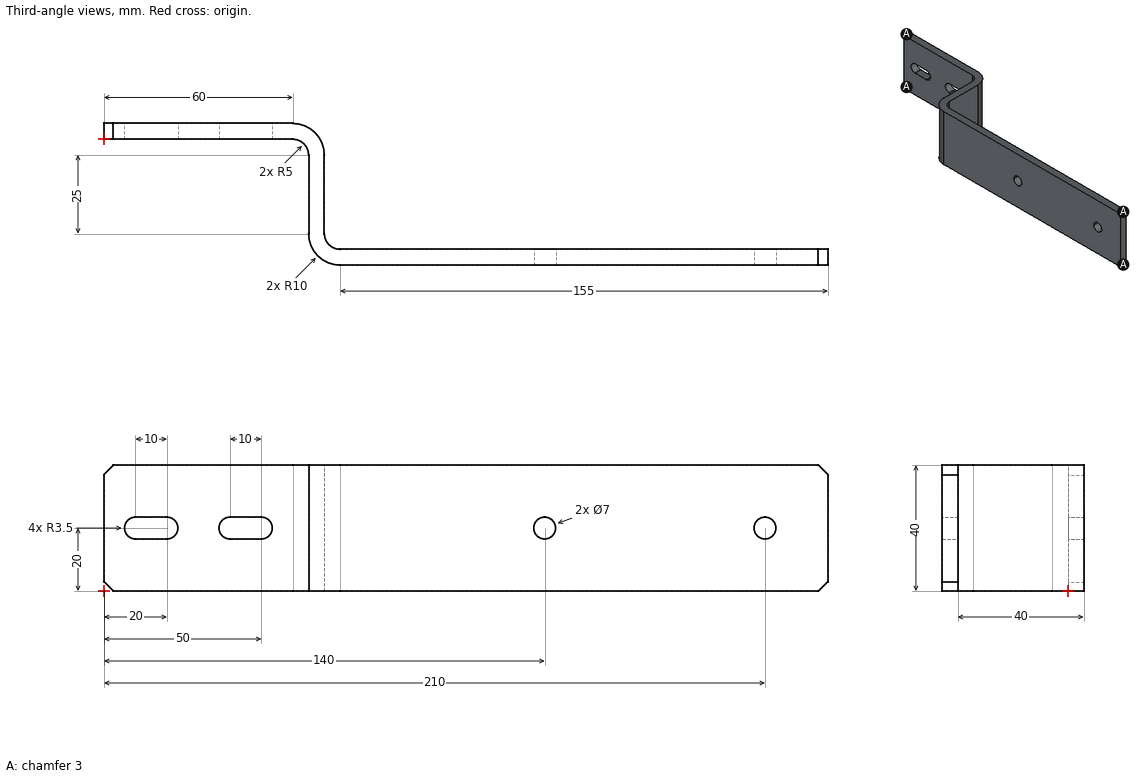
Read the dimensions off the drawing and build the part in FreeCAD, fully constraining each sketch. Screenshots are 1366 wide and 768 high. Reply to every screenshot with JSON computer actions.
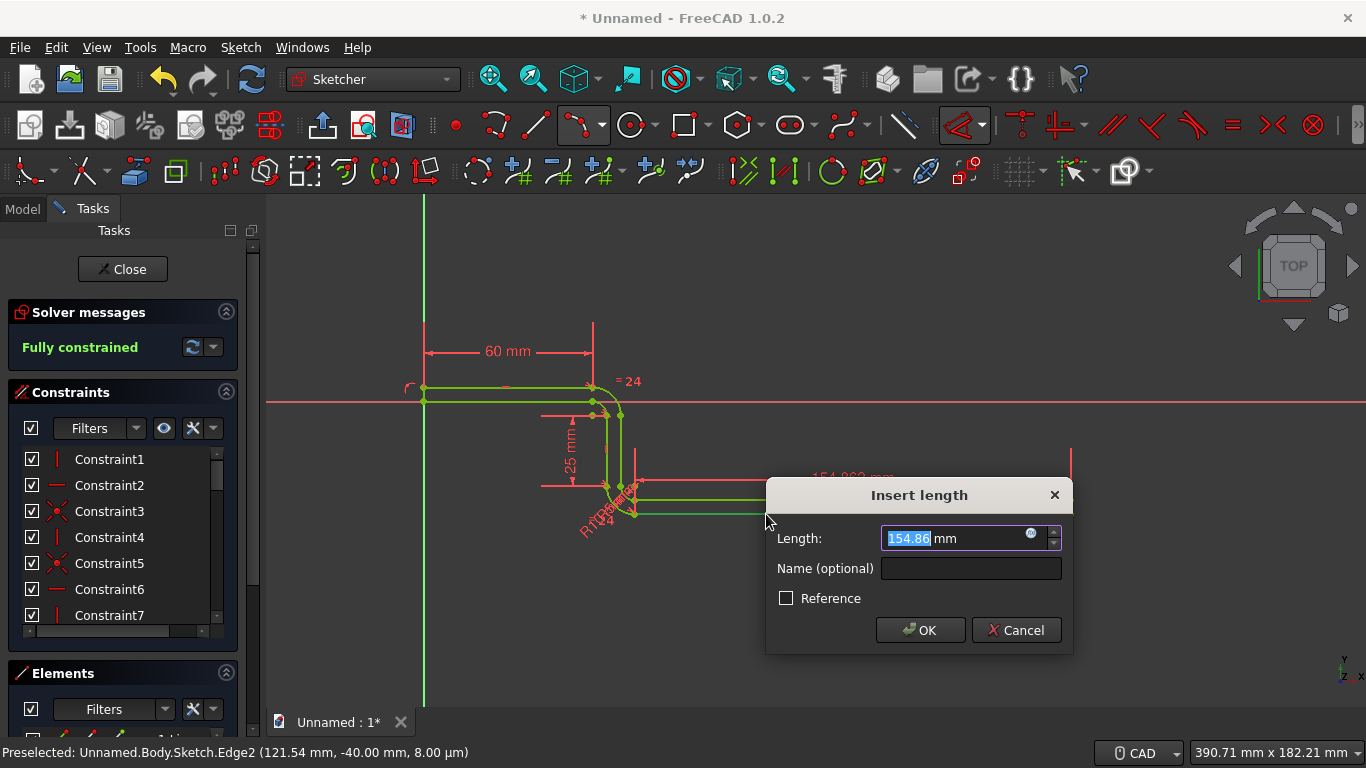
{"action": "type", "text": "155"}
{"action": "key", "text": "Return"}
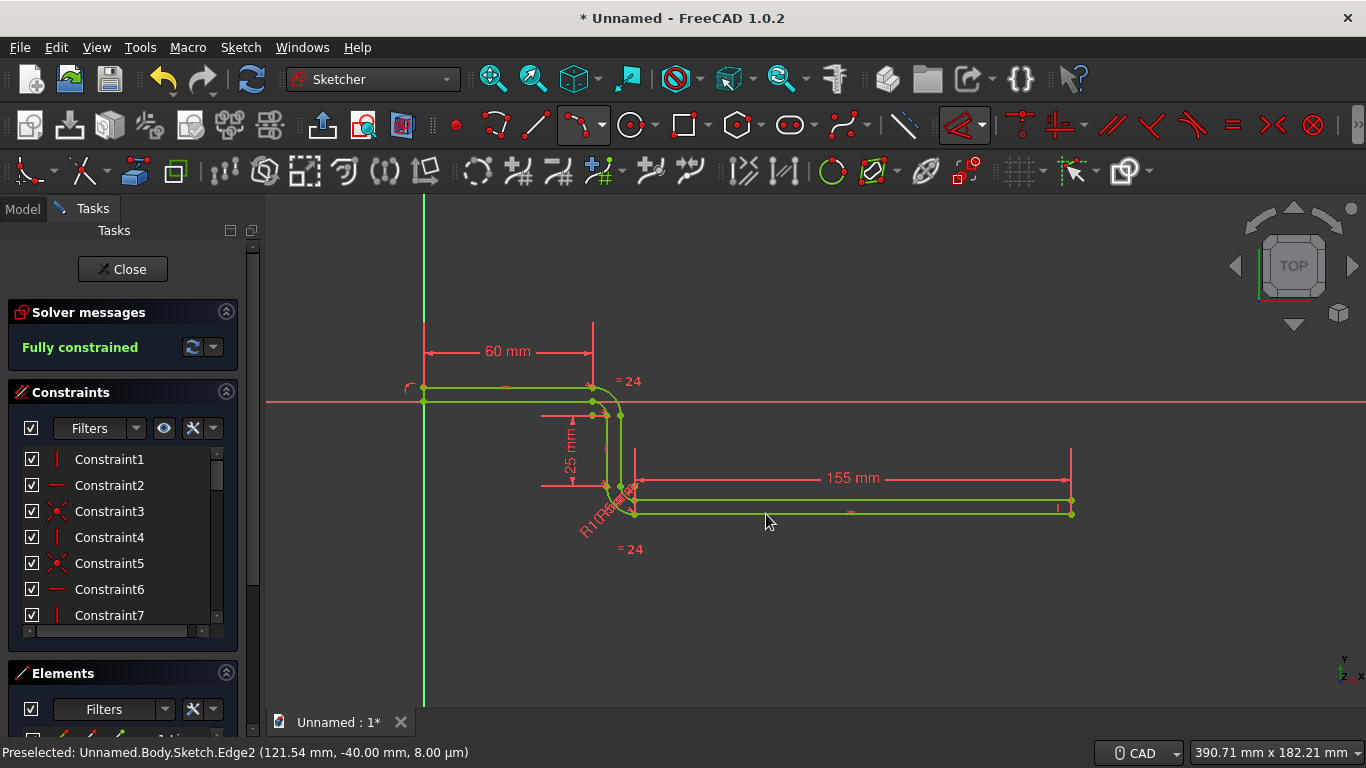
{"action": "left_click", "coordinate": [123, 269]}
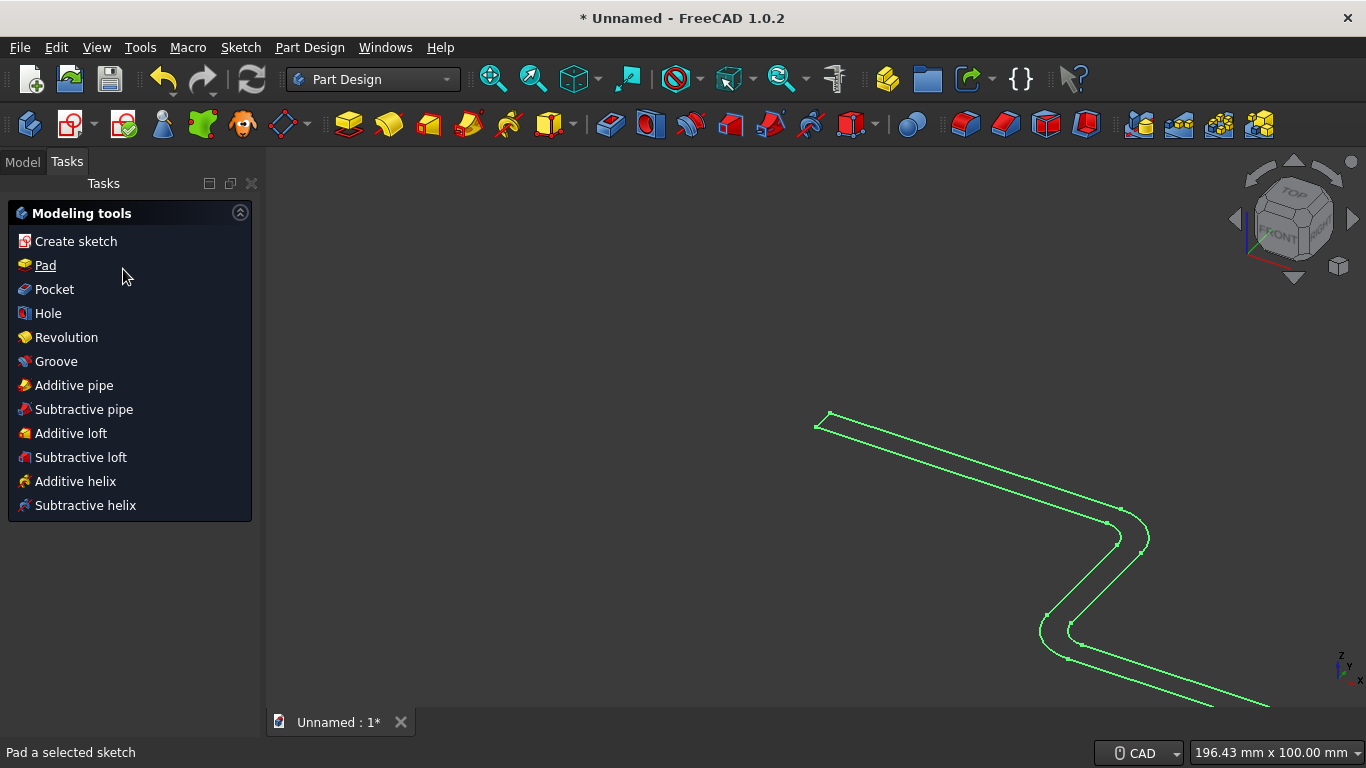
{"action": "left_click", "coordinate": [350, 124]}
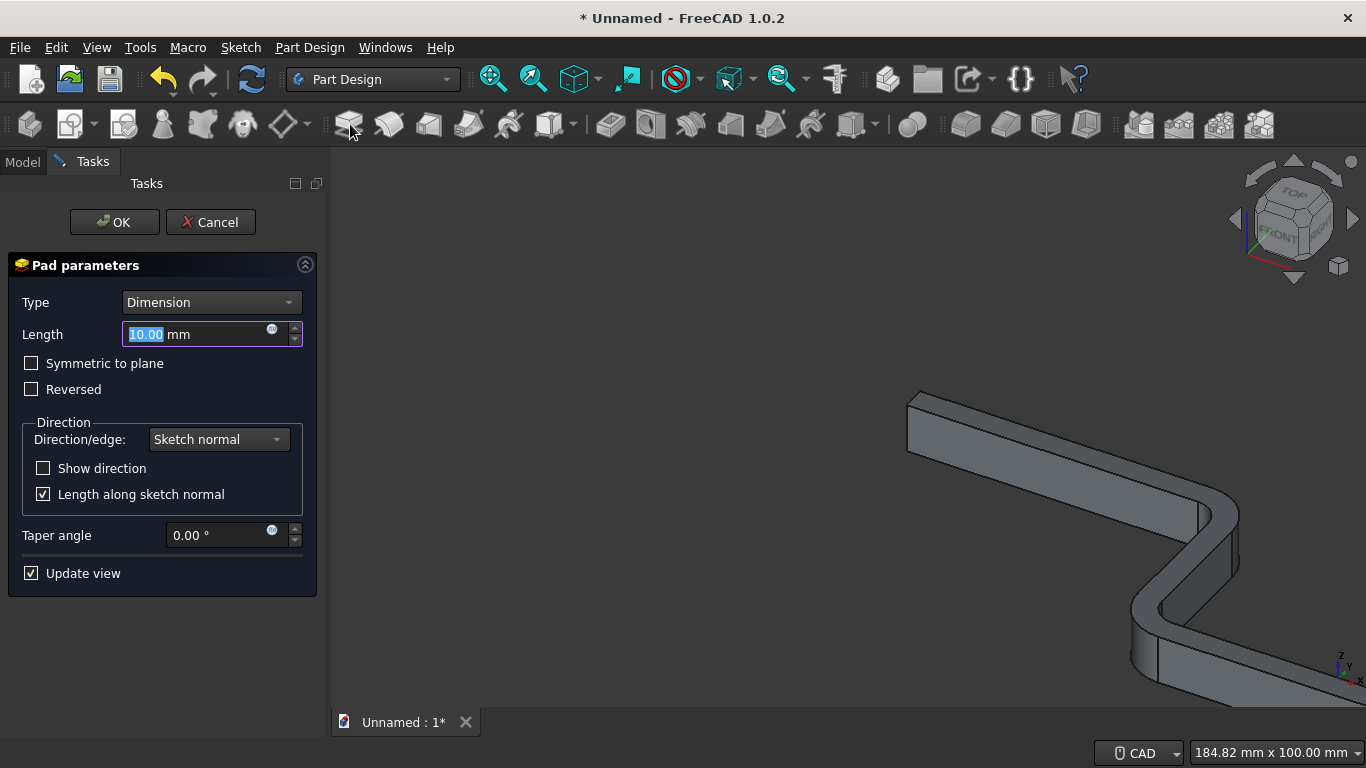
{"action": "type", "text": "40"}
{"action": "key", "text": "Tab"}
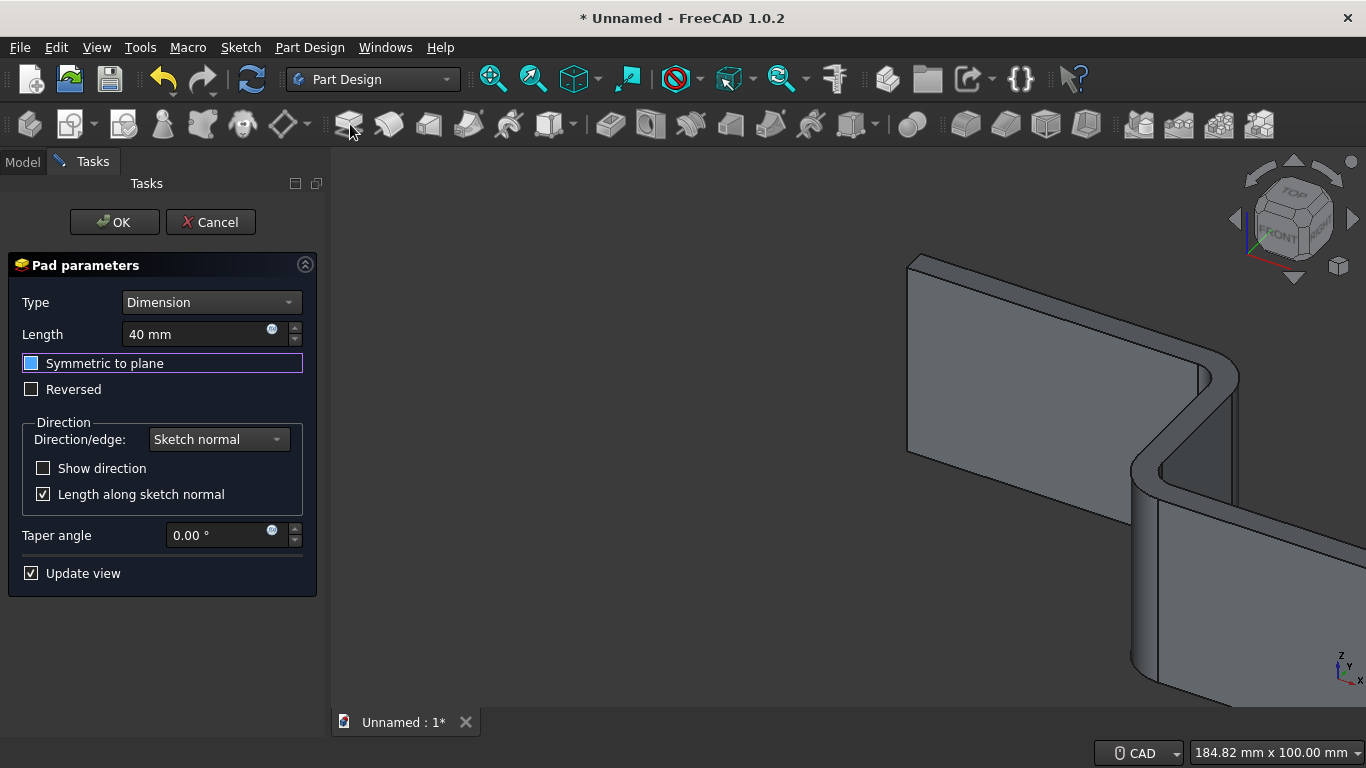
{"action": "left_click", "coordinate": [115, 222]}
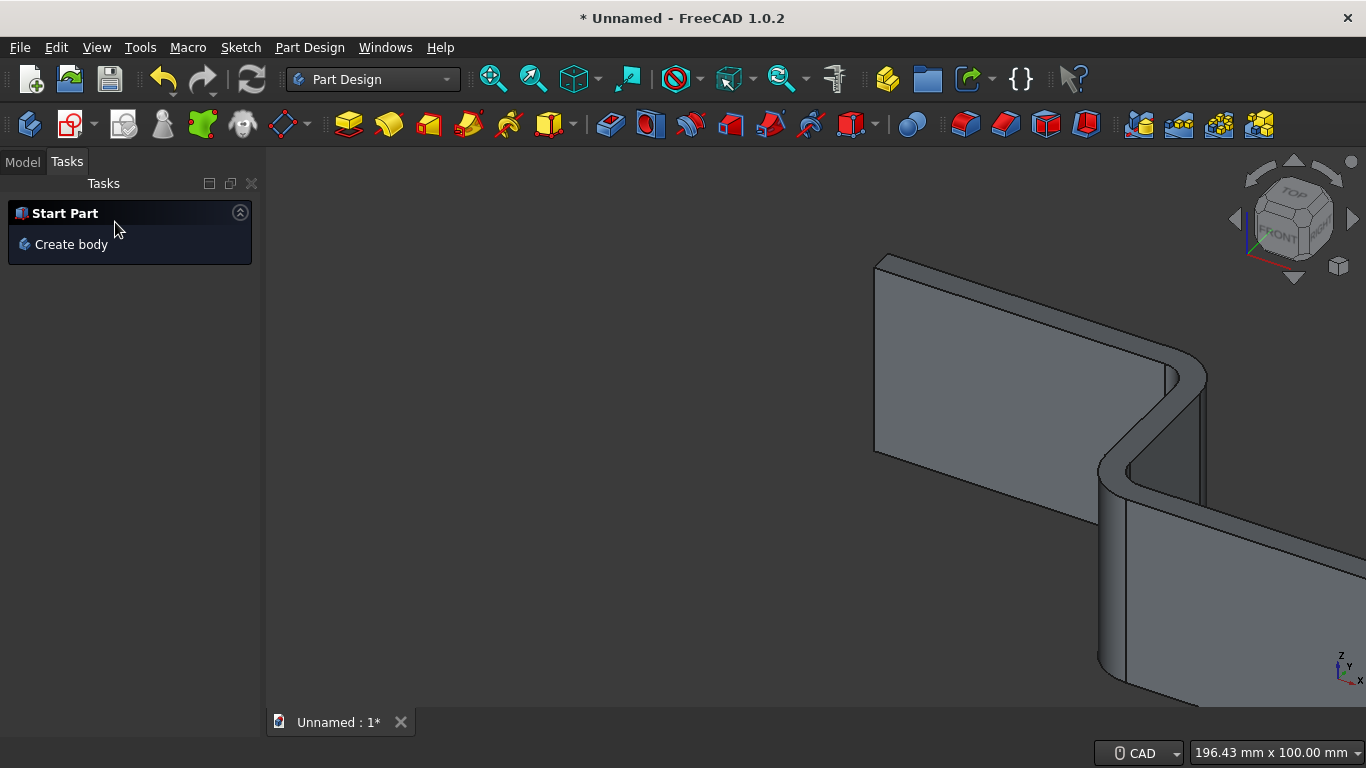
{"action": "left_click", "coordinate": [494, 80]}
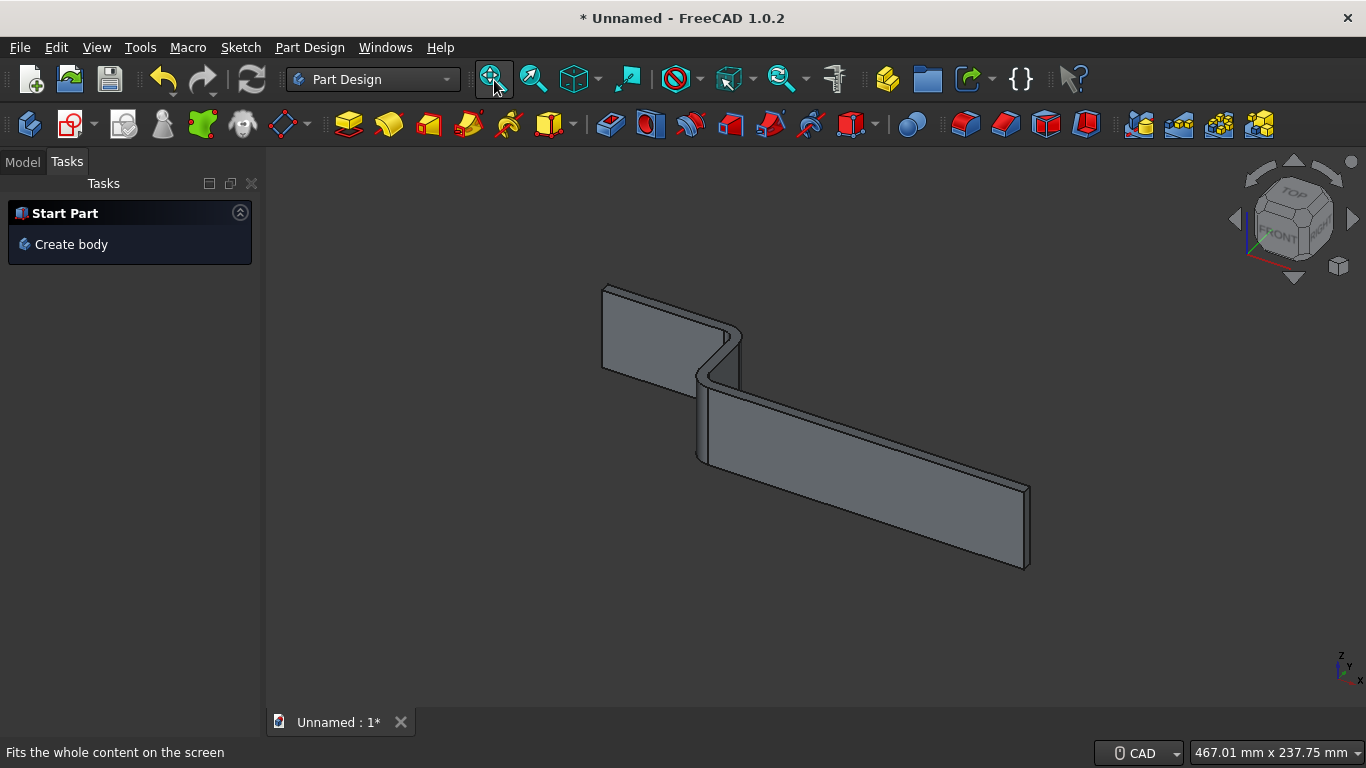
{"action": "key", "text": "4"}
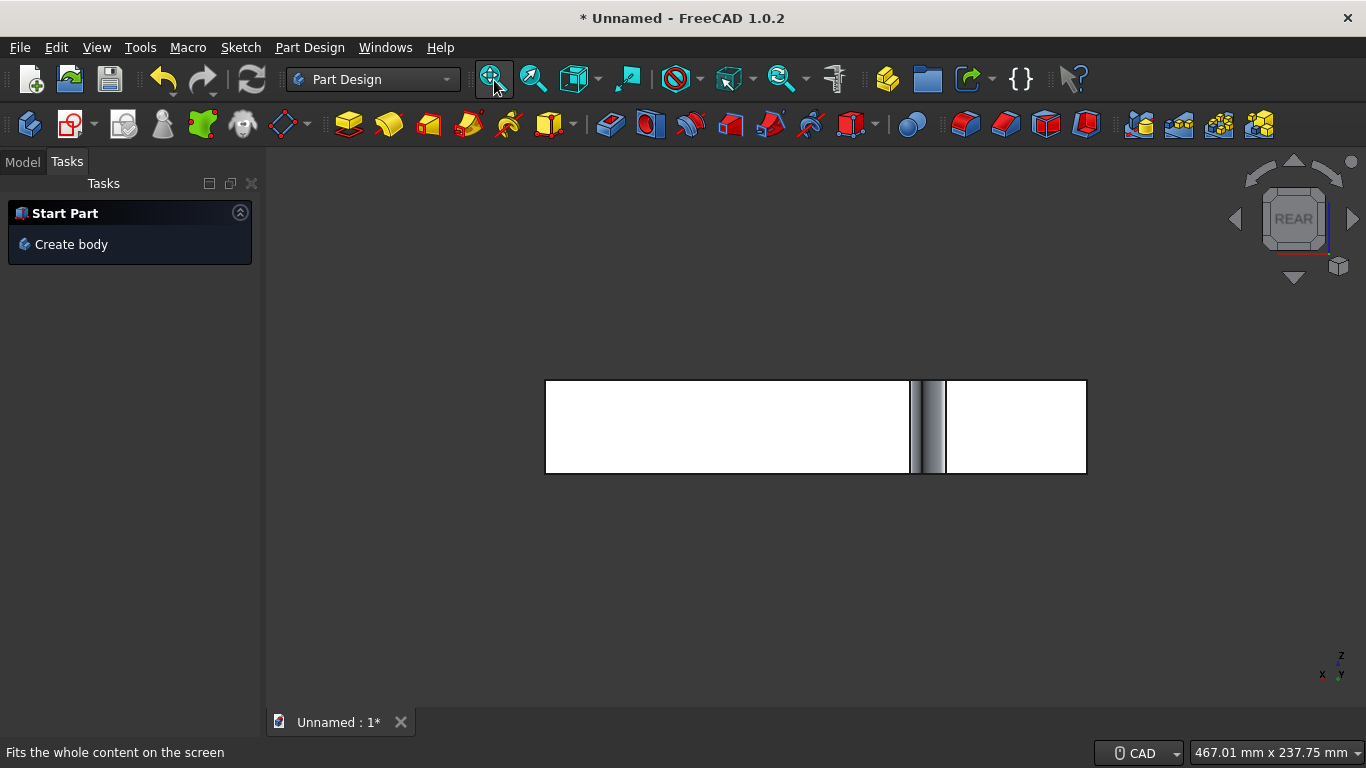
{"action": "left_click", "coordinate": [996, 426]}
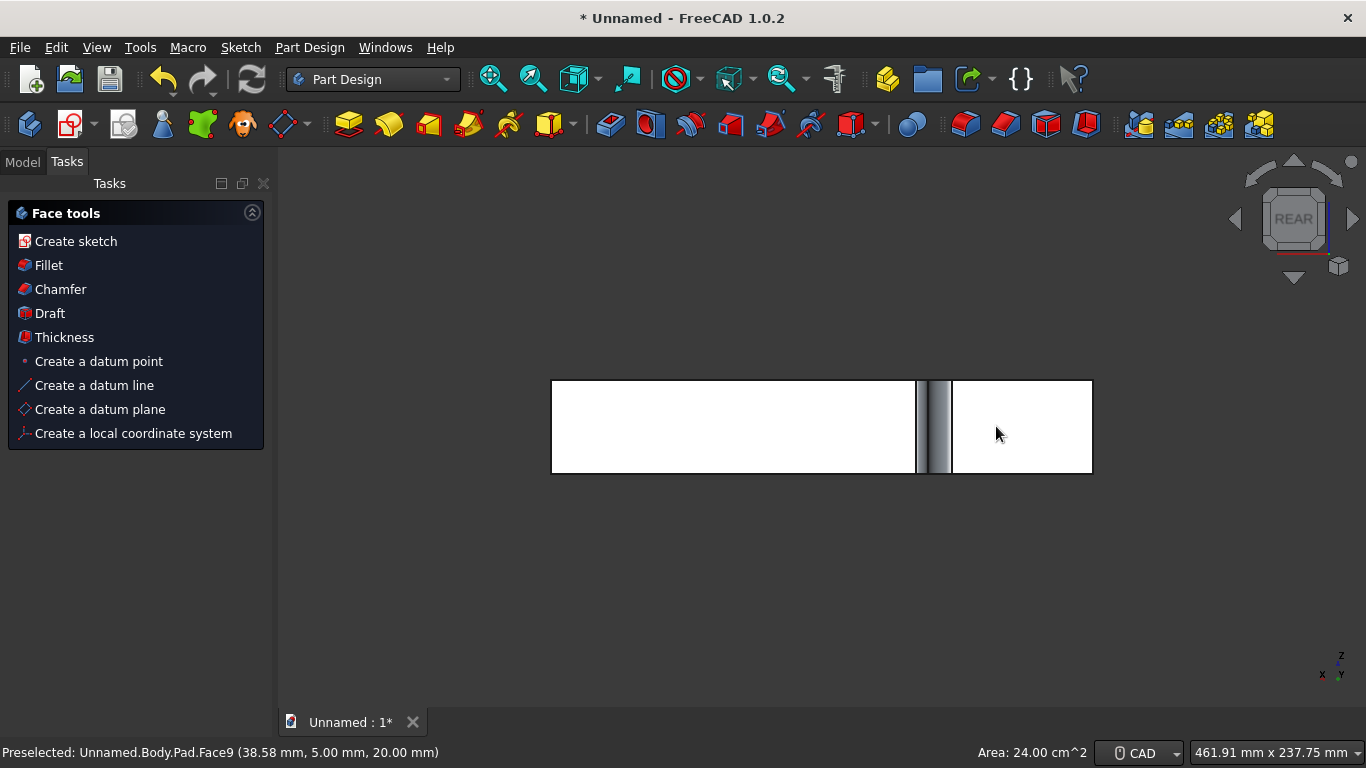
{"action": "left_click", "coordinate": [70, 124]}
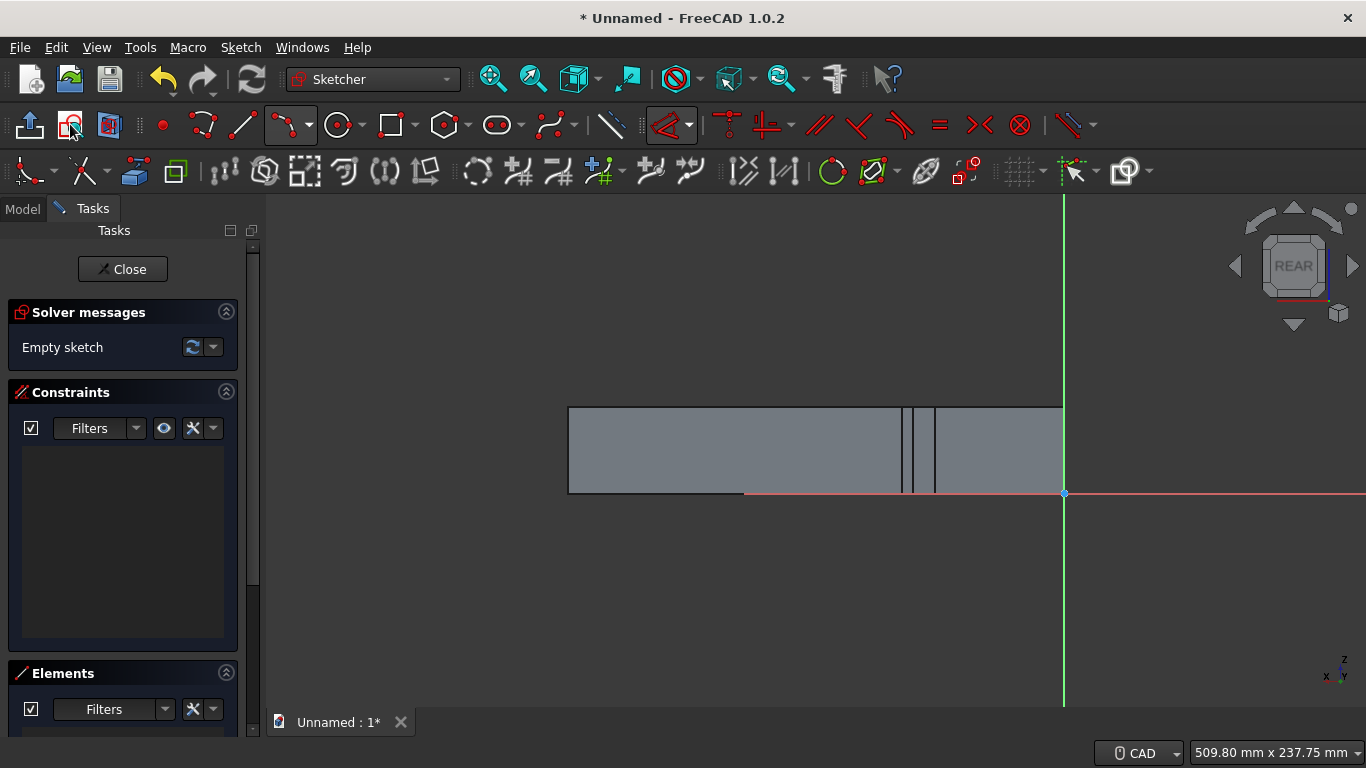
{"action": "scroll", "coordinate": [1058, 472], "scroll_direction": "up", "scroll_amount": 9}